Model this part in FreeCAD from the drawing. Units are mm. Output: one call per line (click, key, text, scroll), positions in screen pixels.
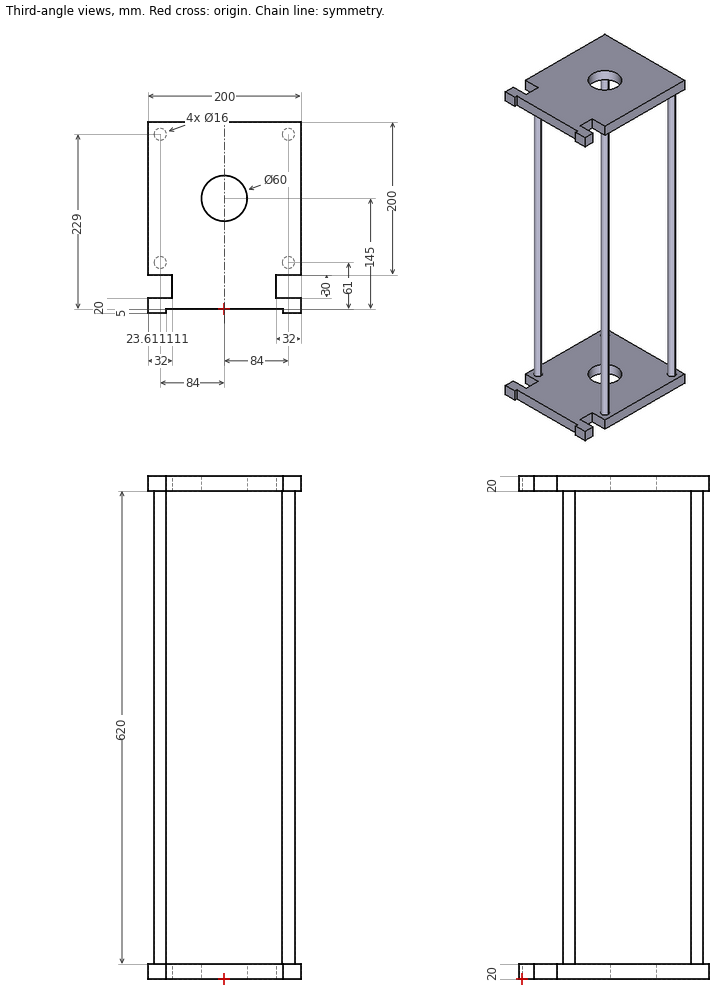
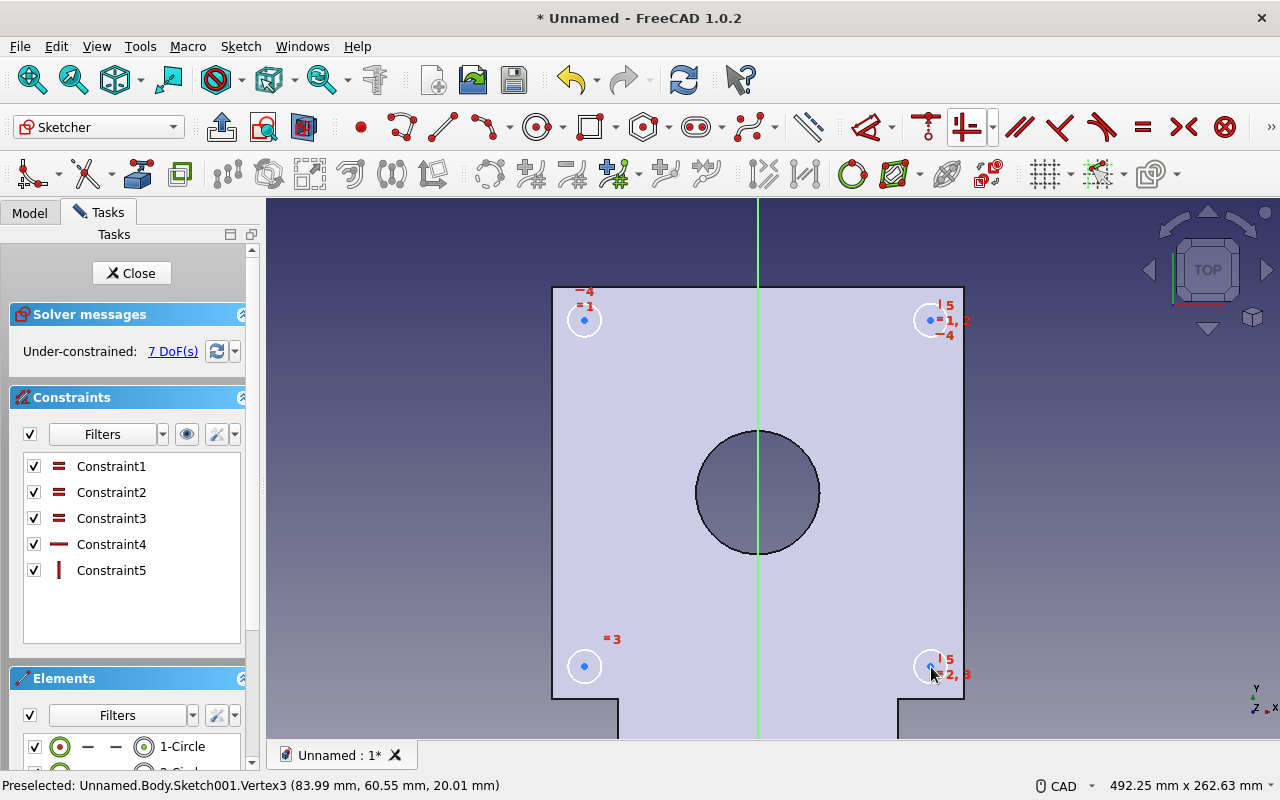
click(585, 320)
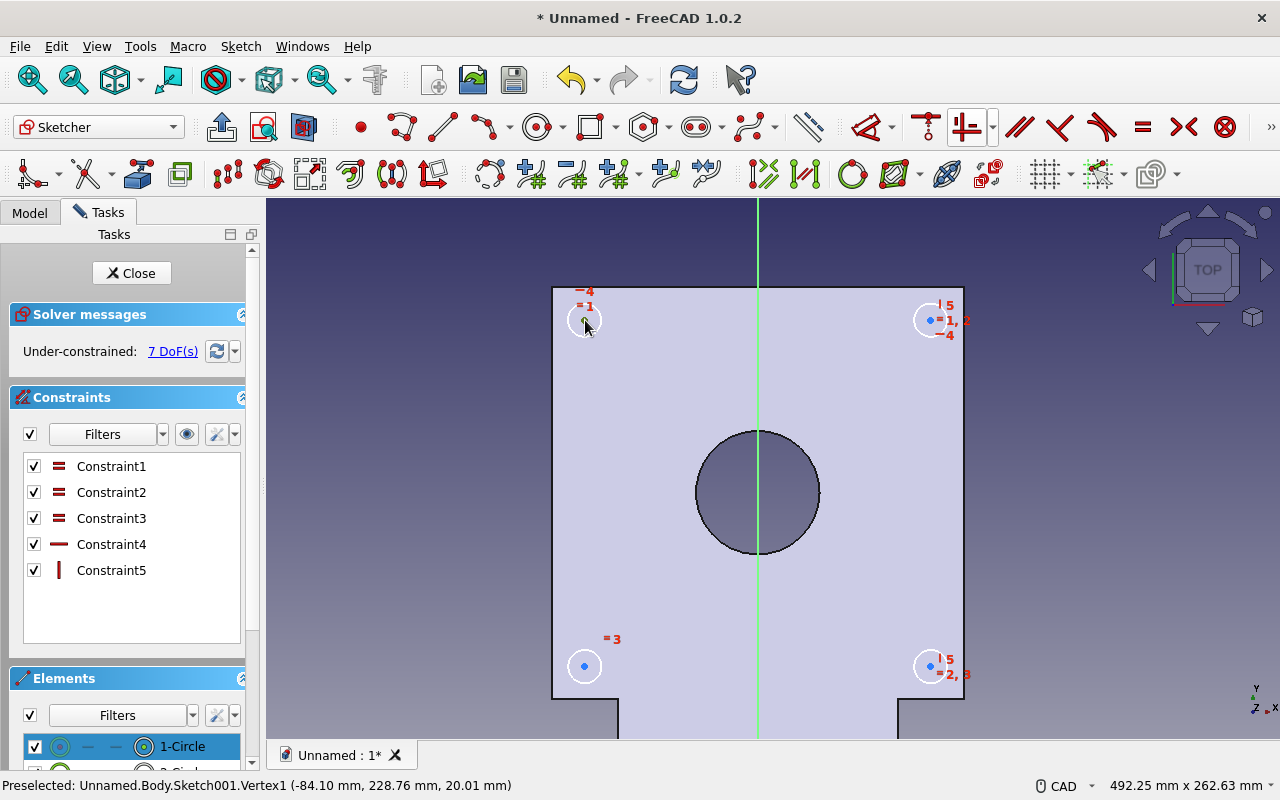
click(585, 667)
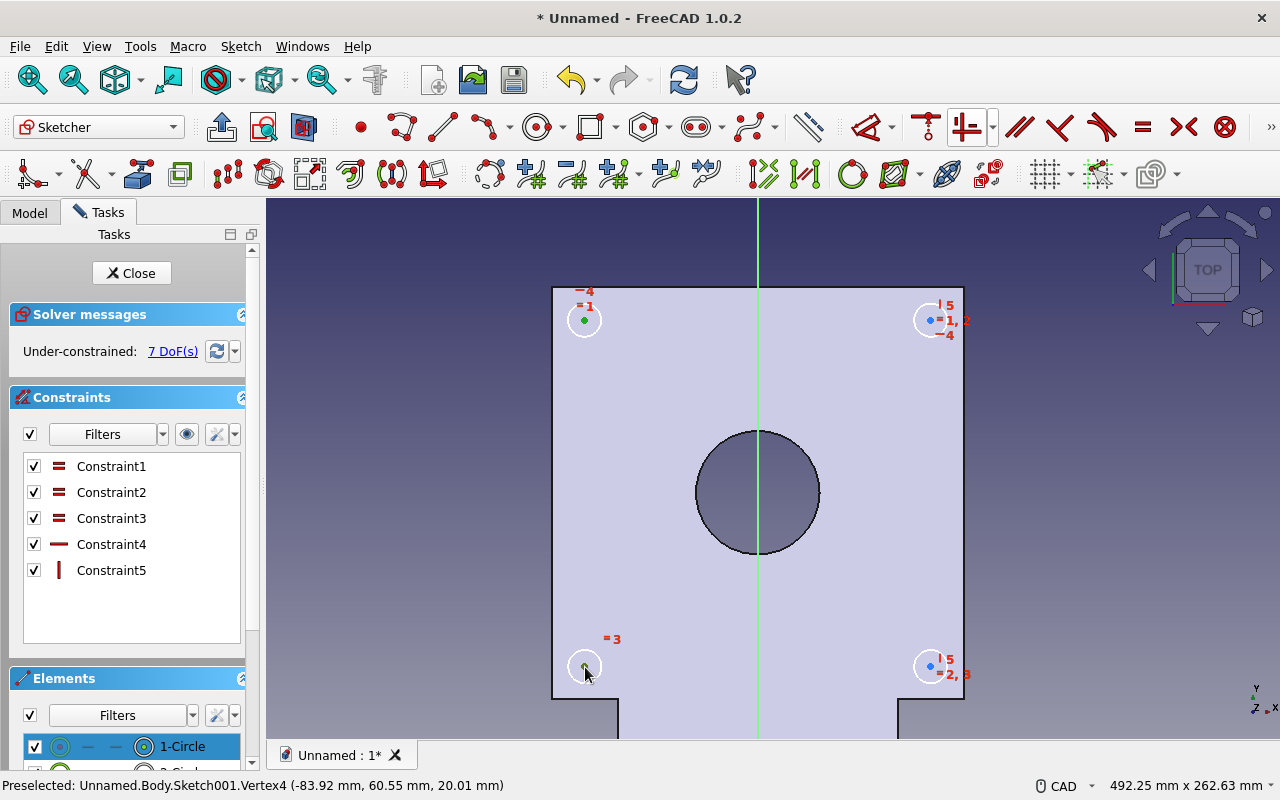
key(v)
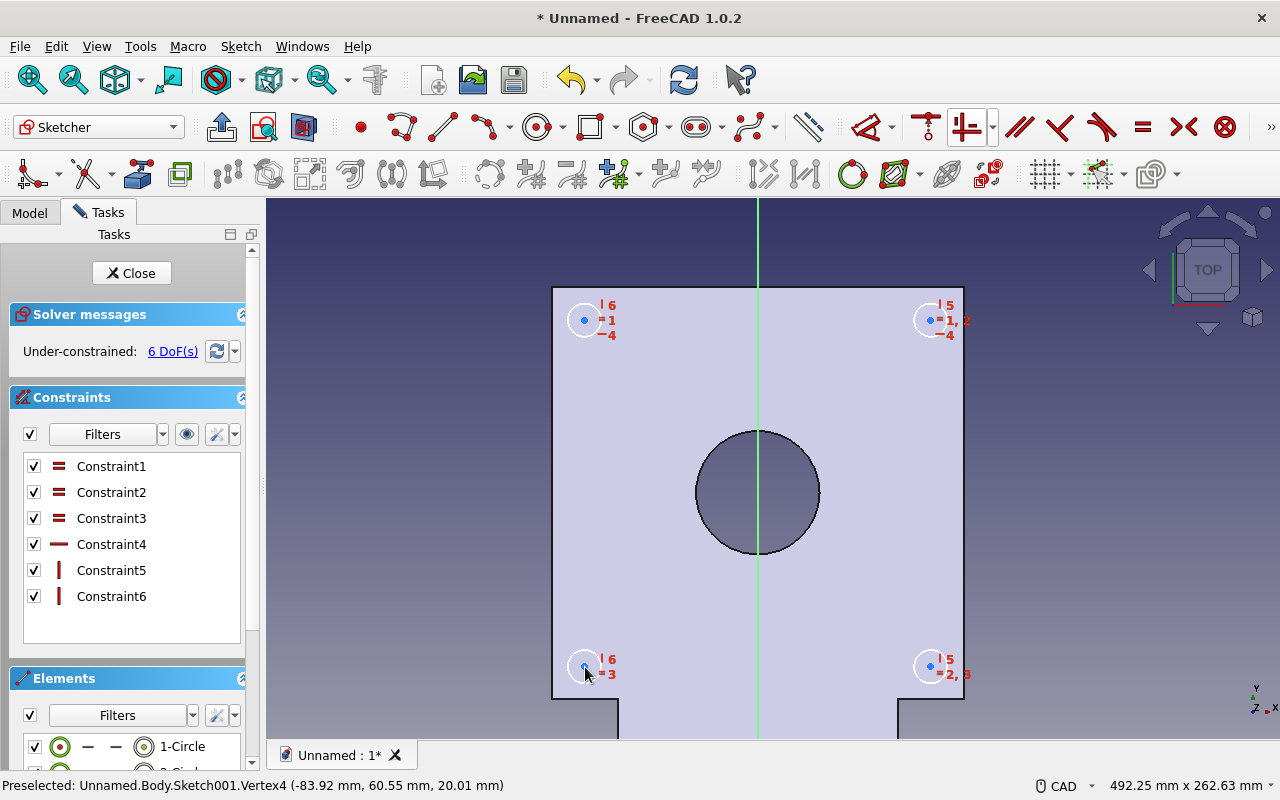
click(931, 667)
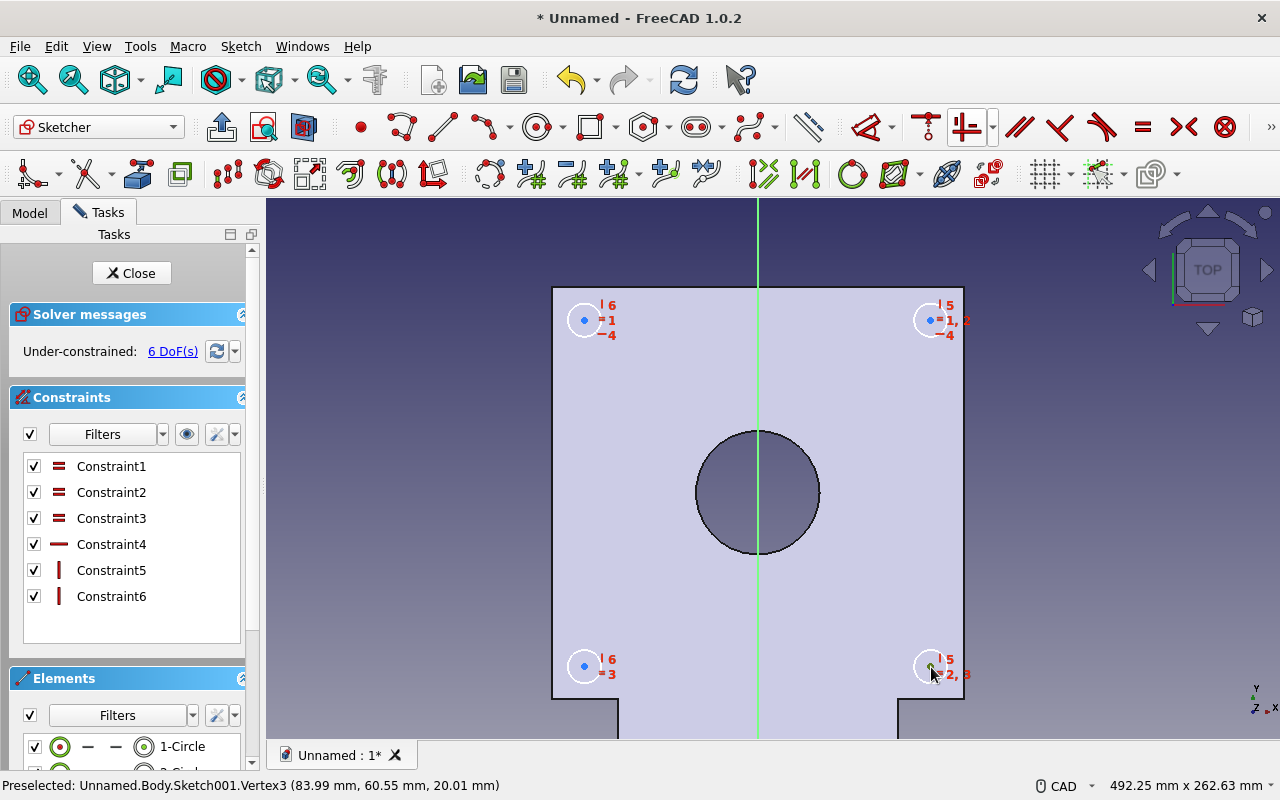
click(585, 667)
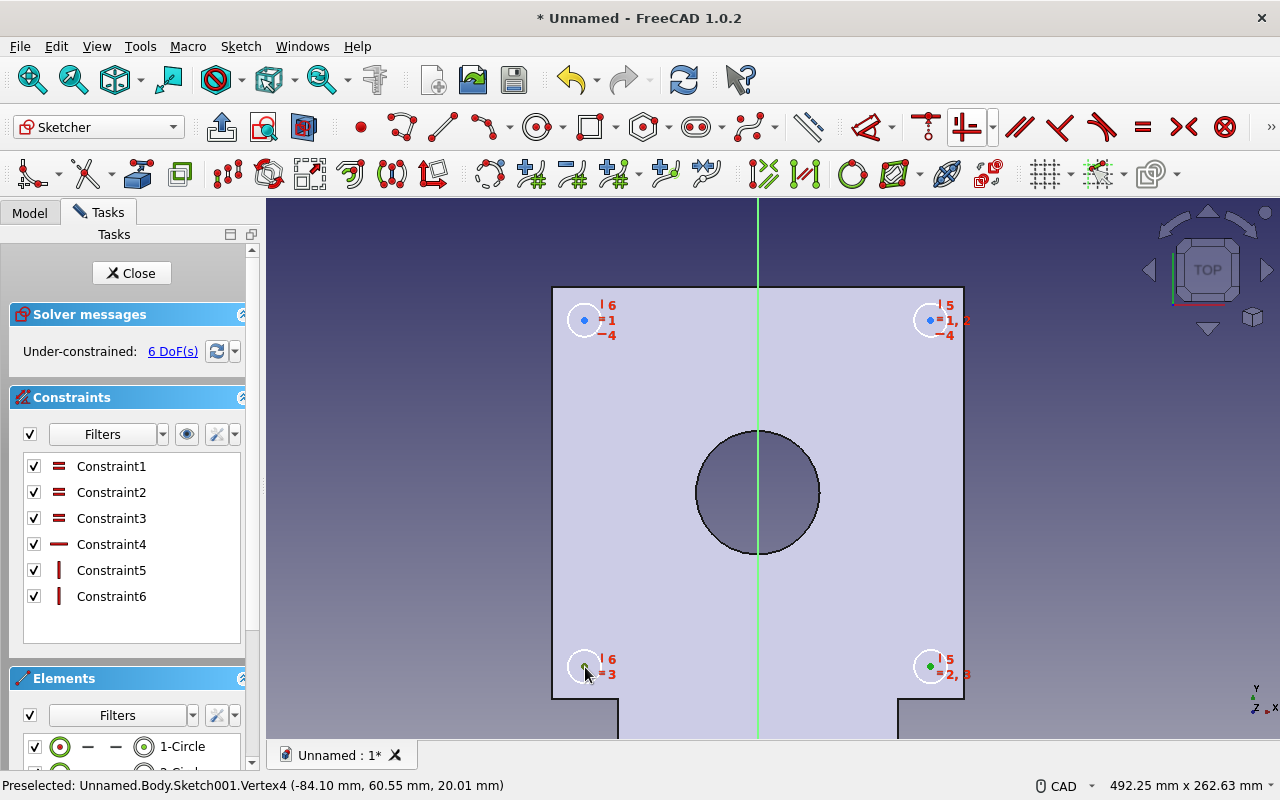
key(h)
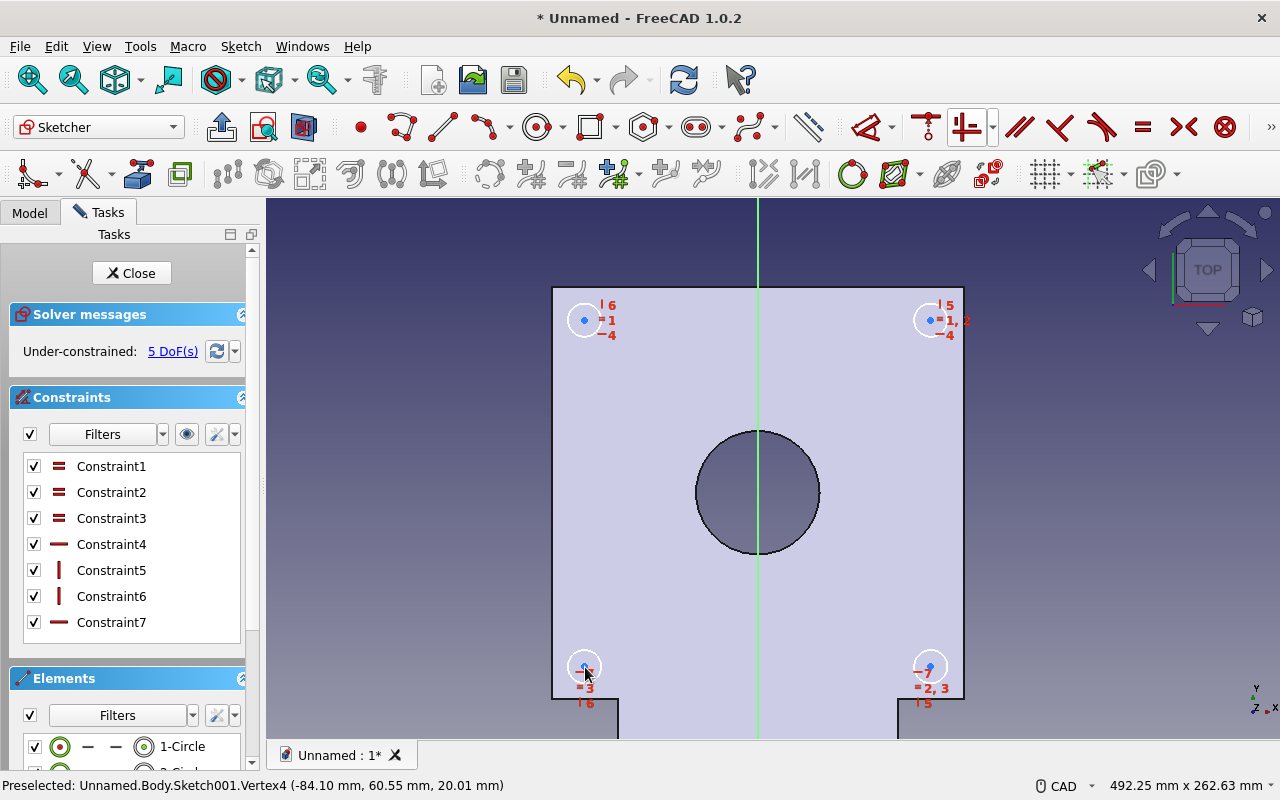
click(866, 128)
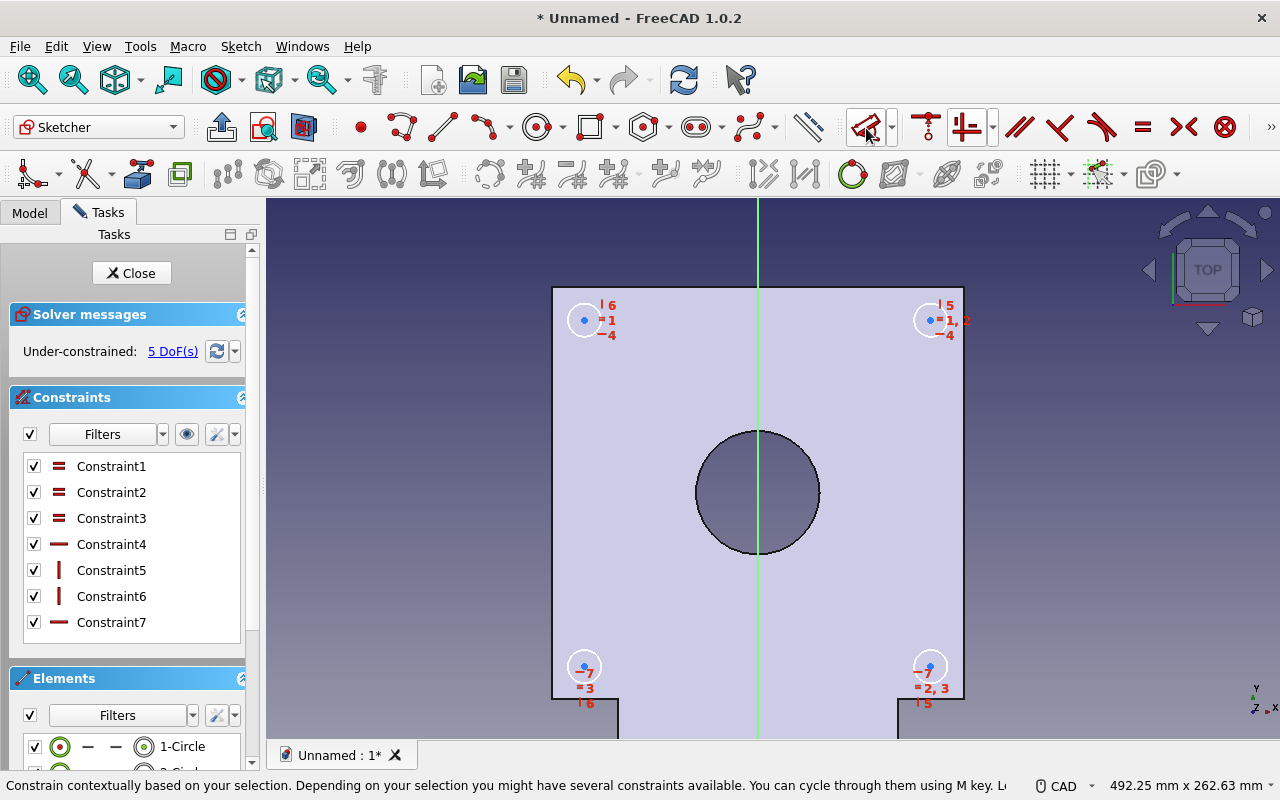
click(596, 308)
click(618, 285)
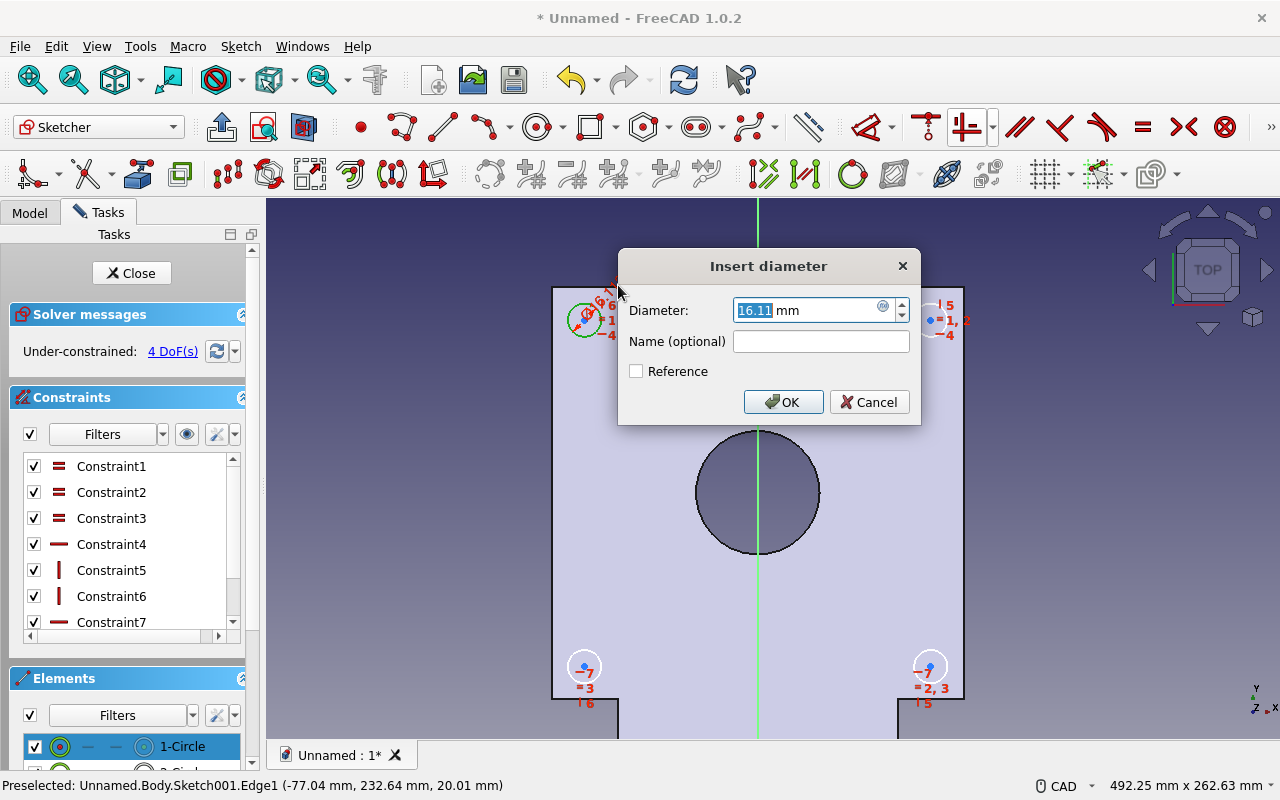
text(16)
key(Return)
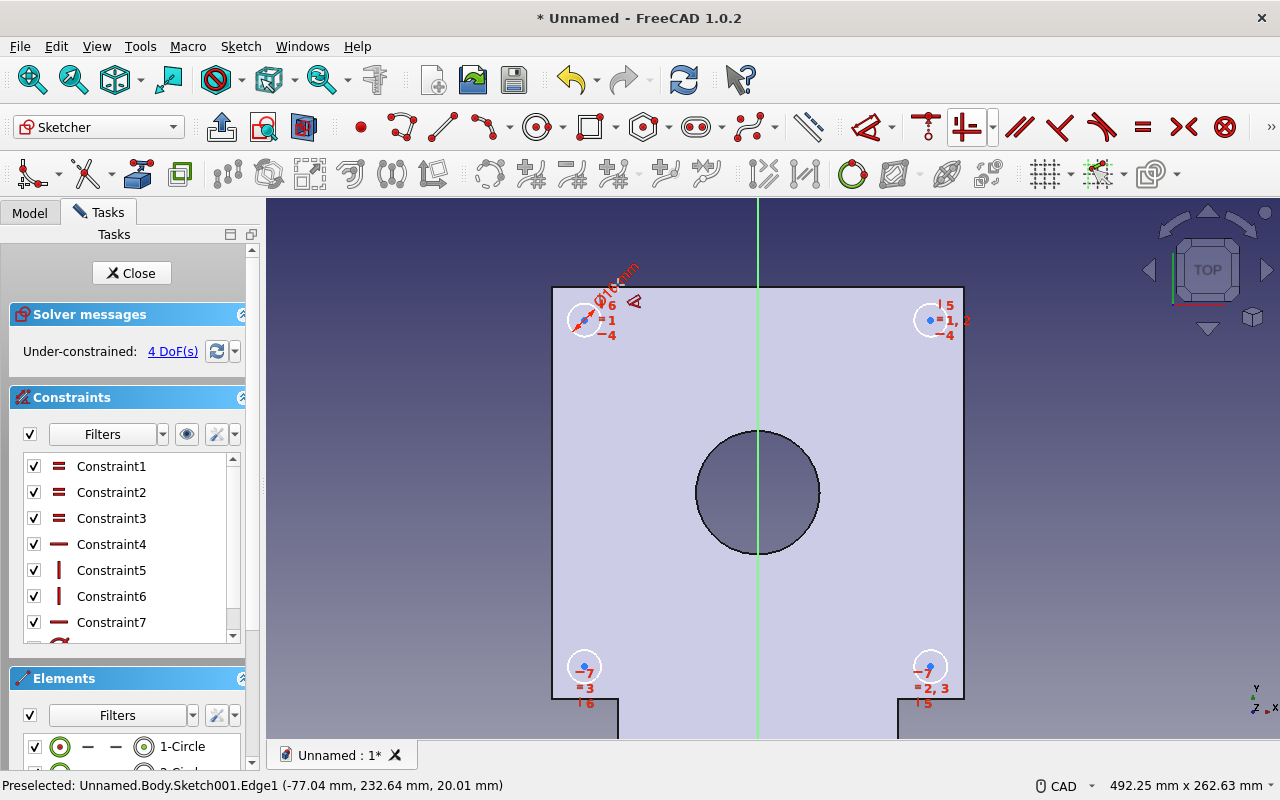
click(585, 320)
click(711, 286)